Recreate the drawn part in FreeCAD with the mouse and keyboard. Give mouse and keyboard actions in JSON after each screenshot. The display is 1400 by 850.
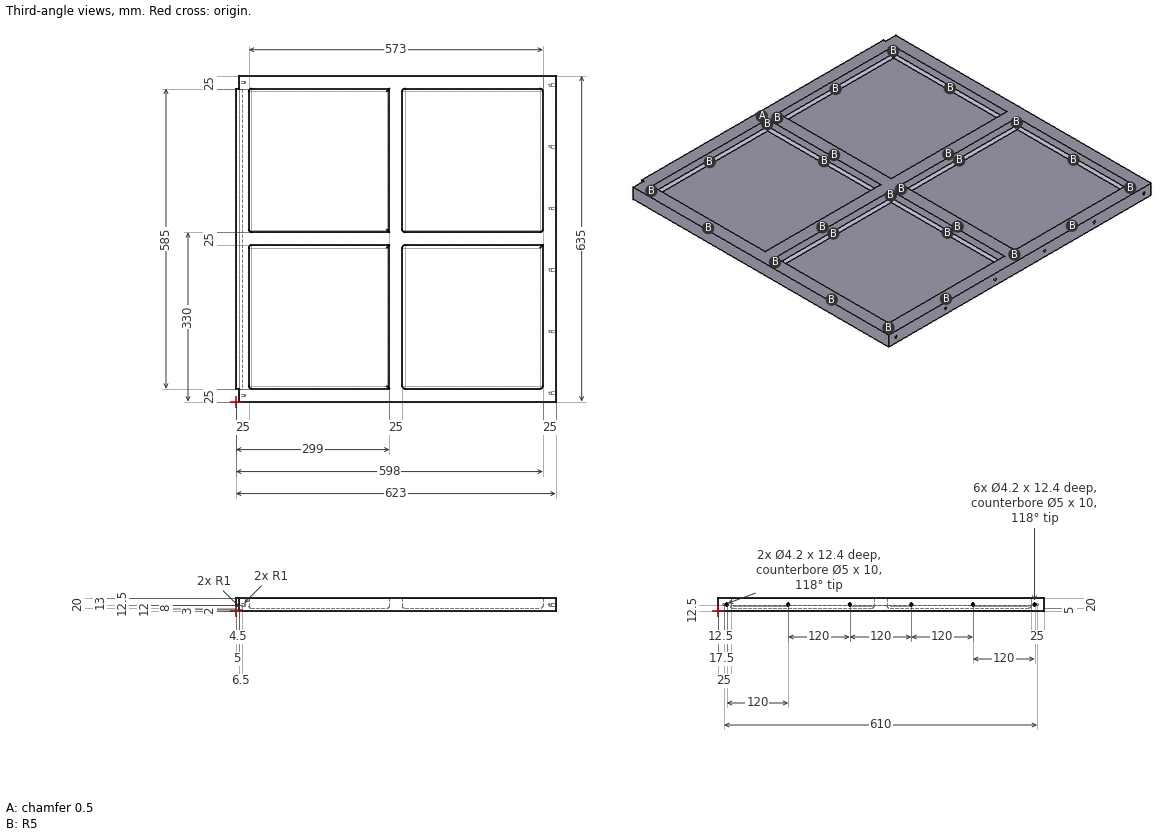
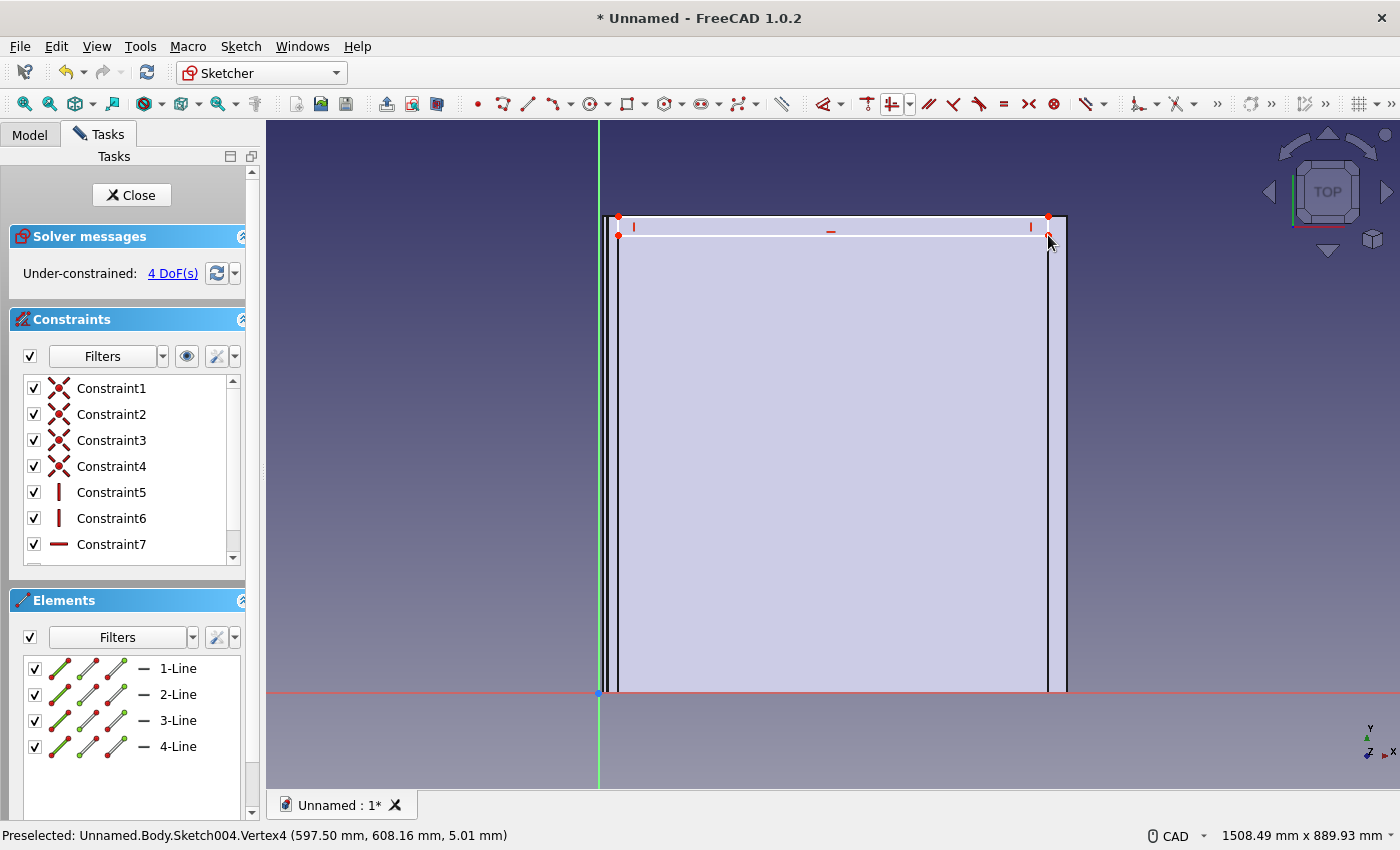
{"action": "left_click", "coordinate": [822, 104]}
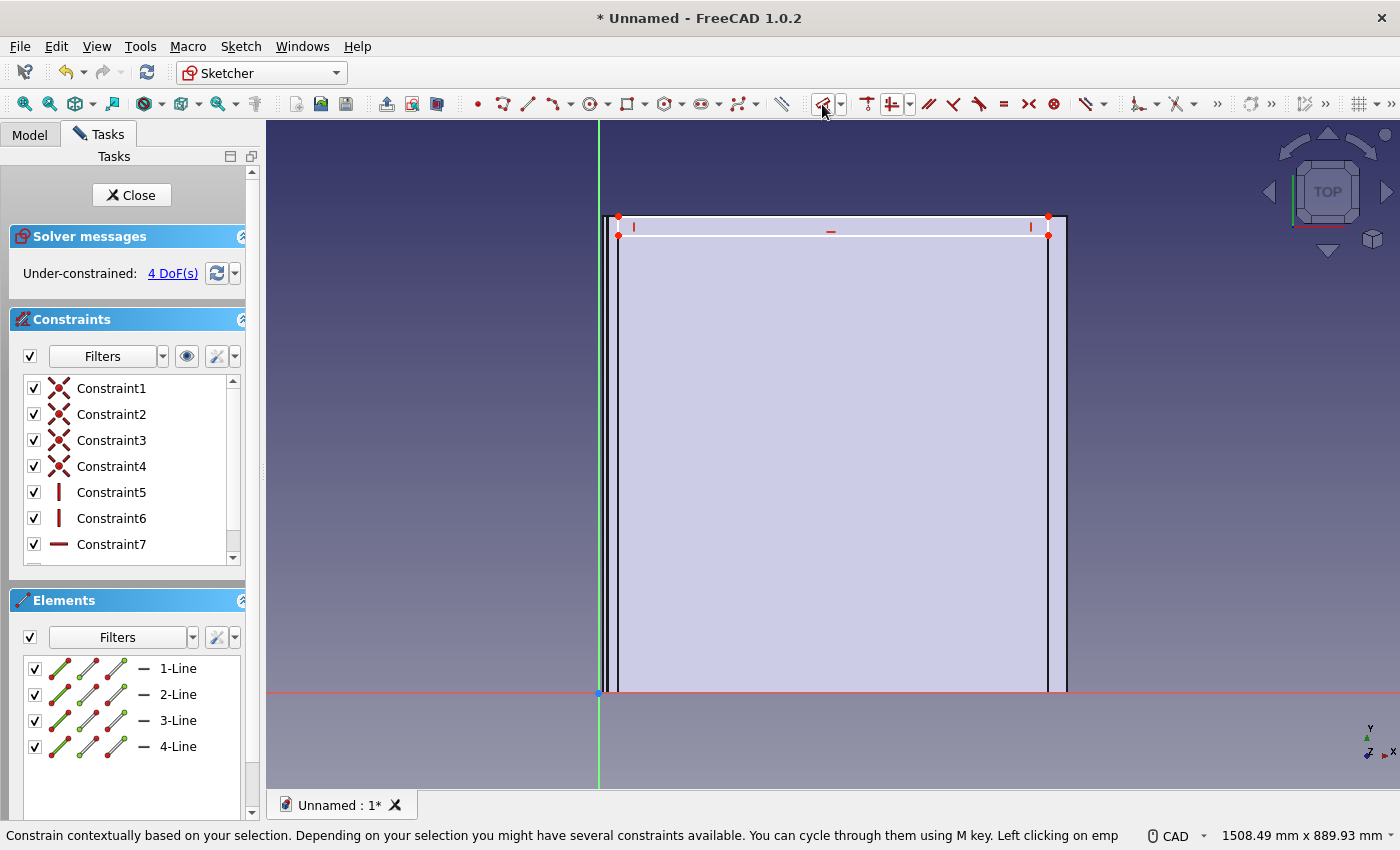
{"action": "scroll", "coordinate": [618, 227], "scroll_direction": "up", "scroll_amount": 4}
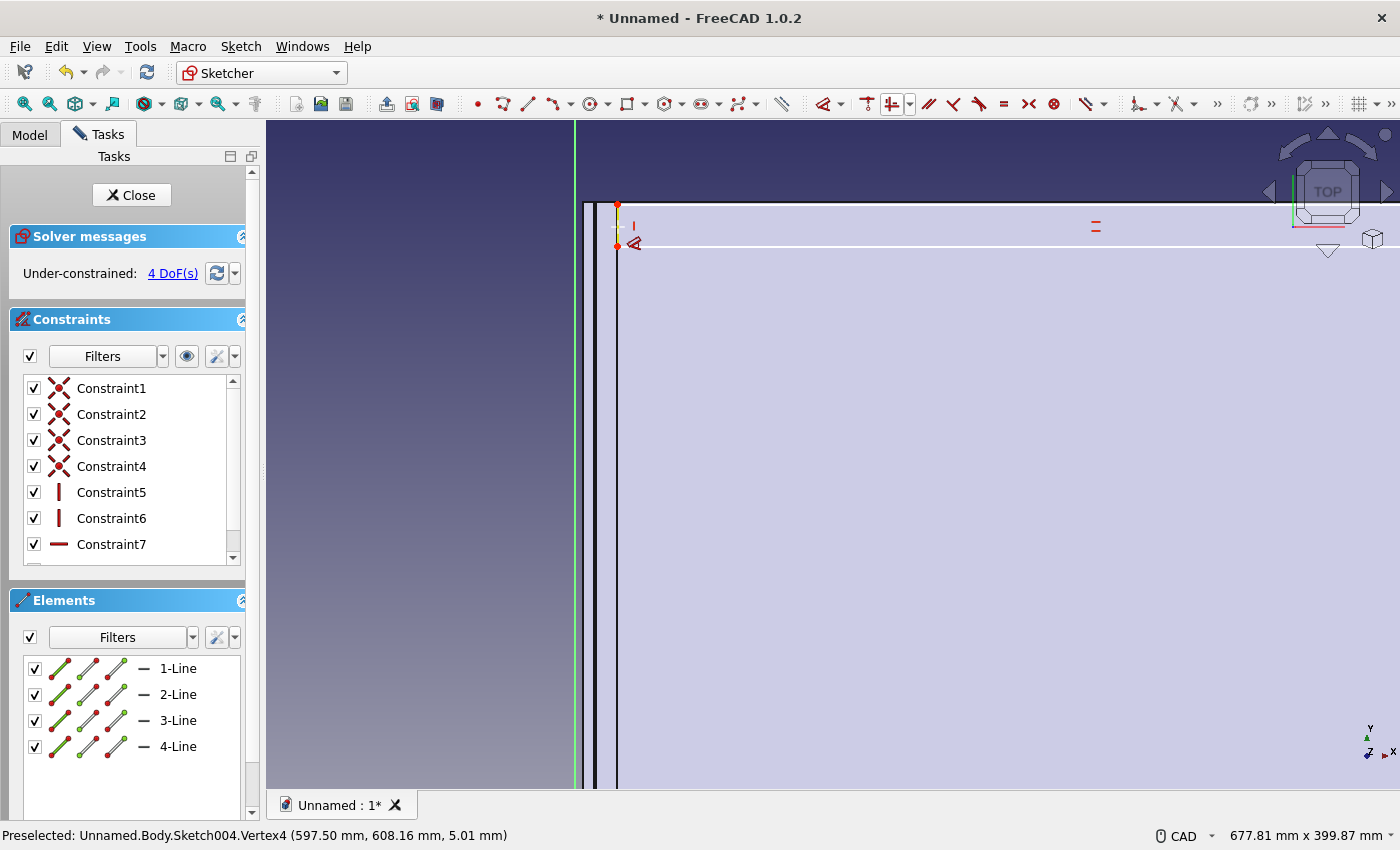
{"action": "left_click", "coordinate": [618, 226]}
{"action": "left_click", "coordinate": [652, 226]}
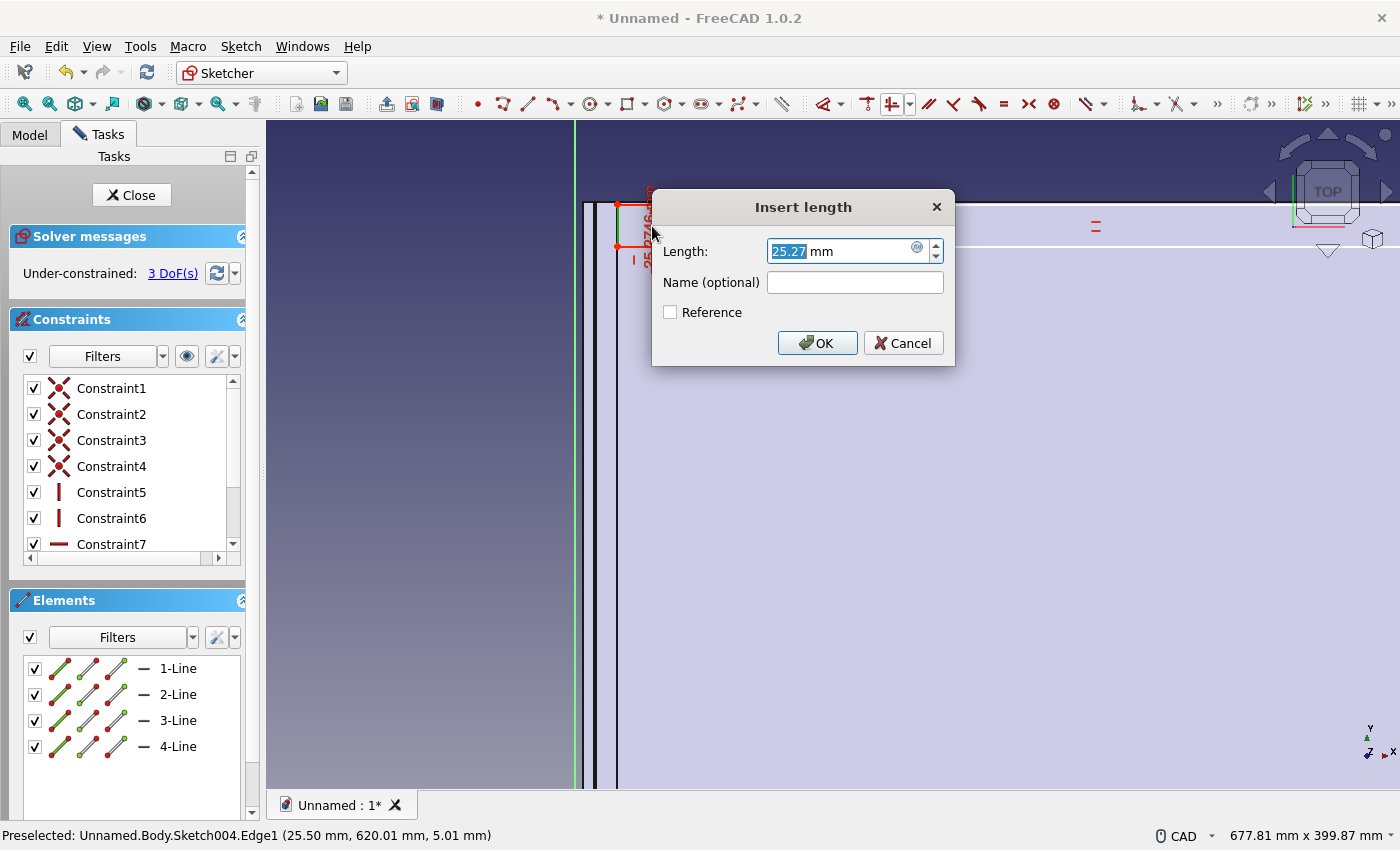
{"action": "type", "text": "25"}
{"action": "key", "text": "Return"}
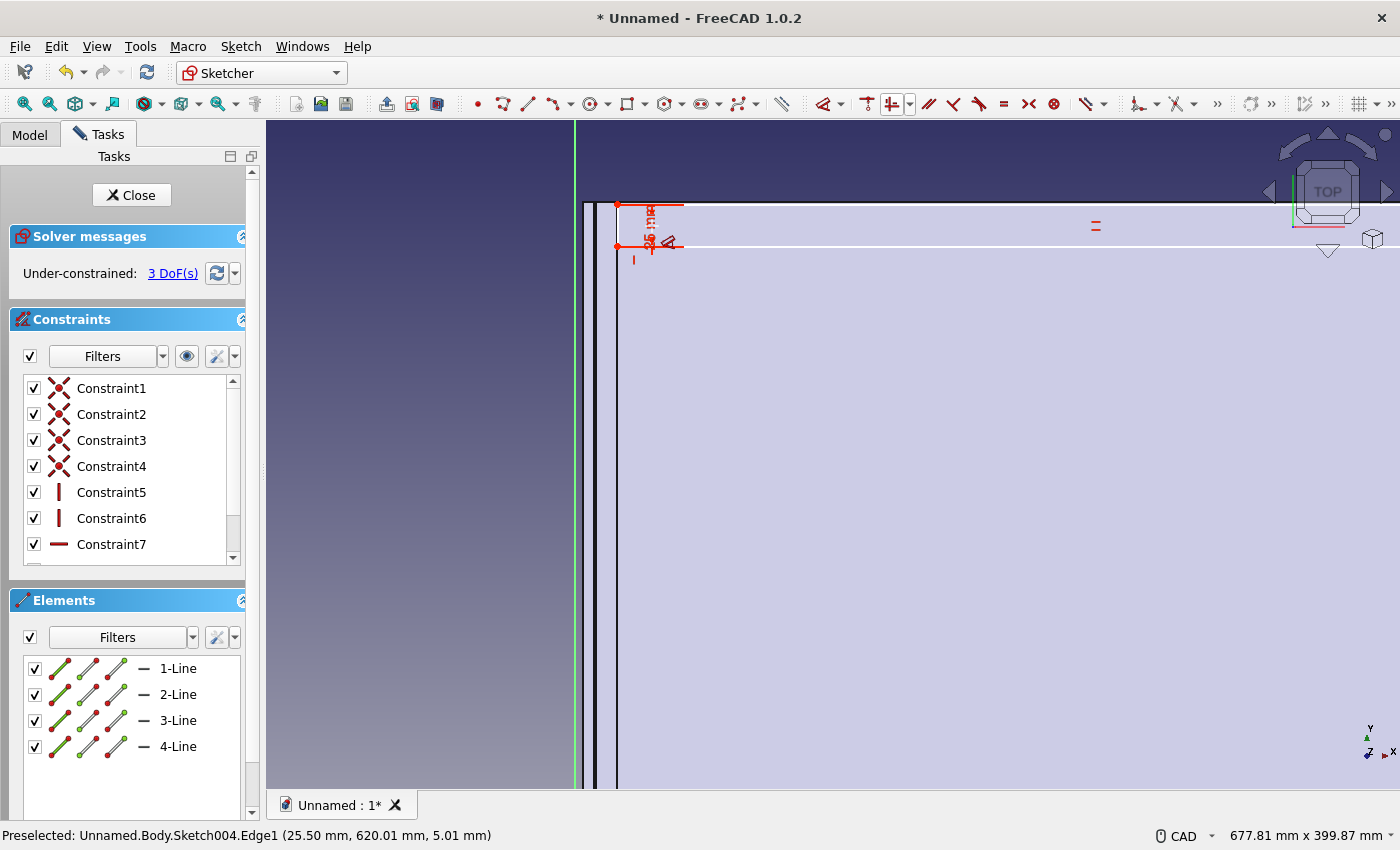
{"action": "left_click", "coordinate": [905, 247]}
{"action": "left_click", "coordinate": [926, 281]}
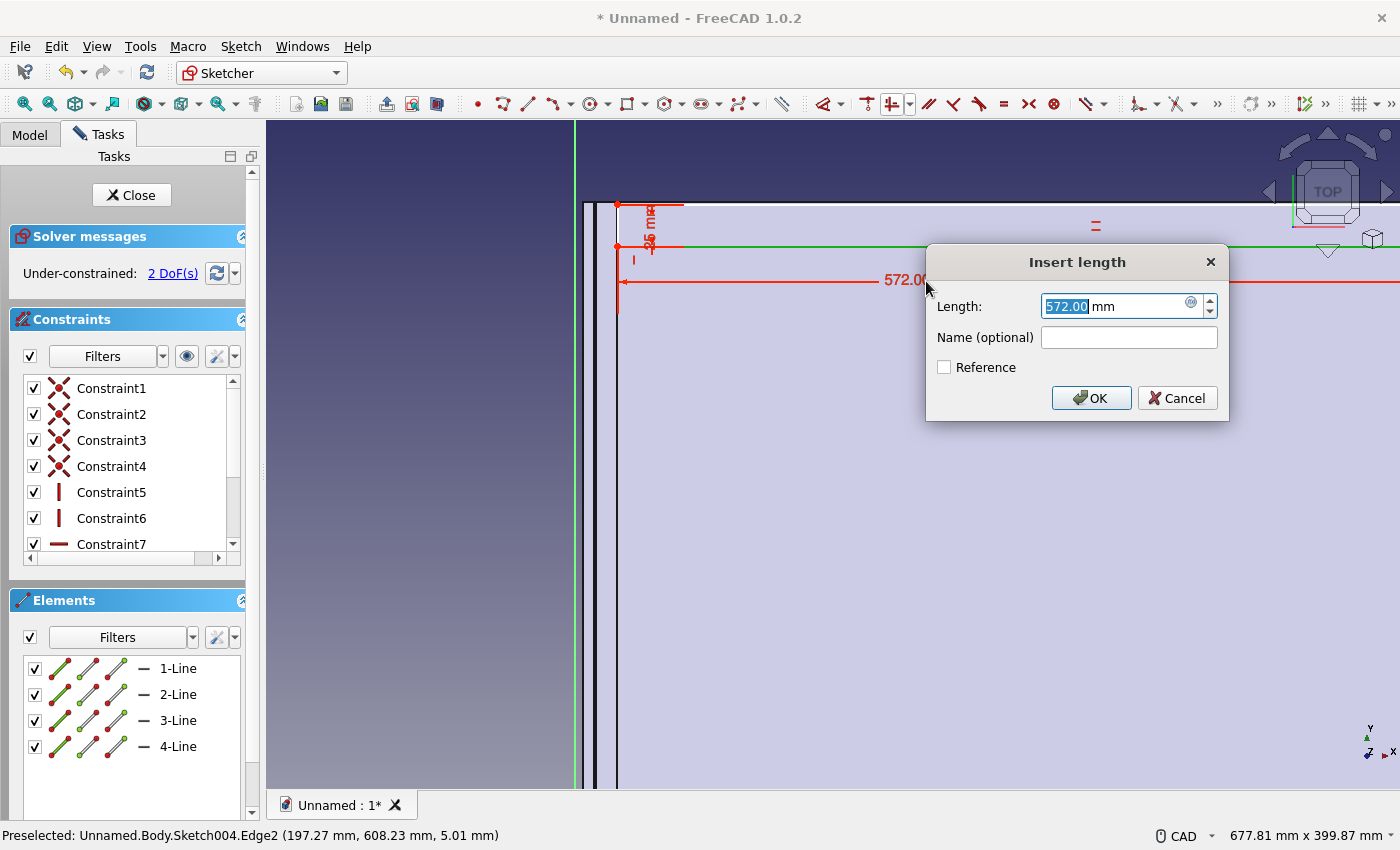
{"action": "type", "text": "573"}
{"action": "key", "text": "Return"}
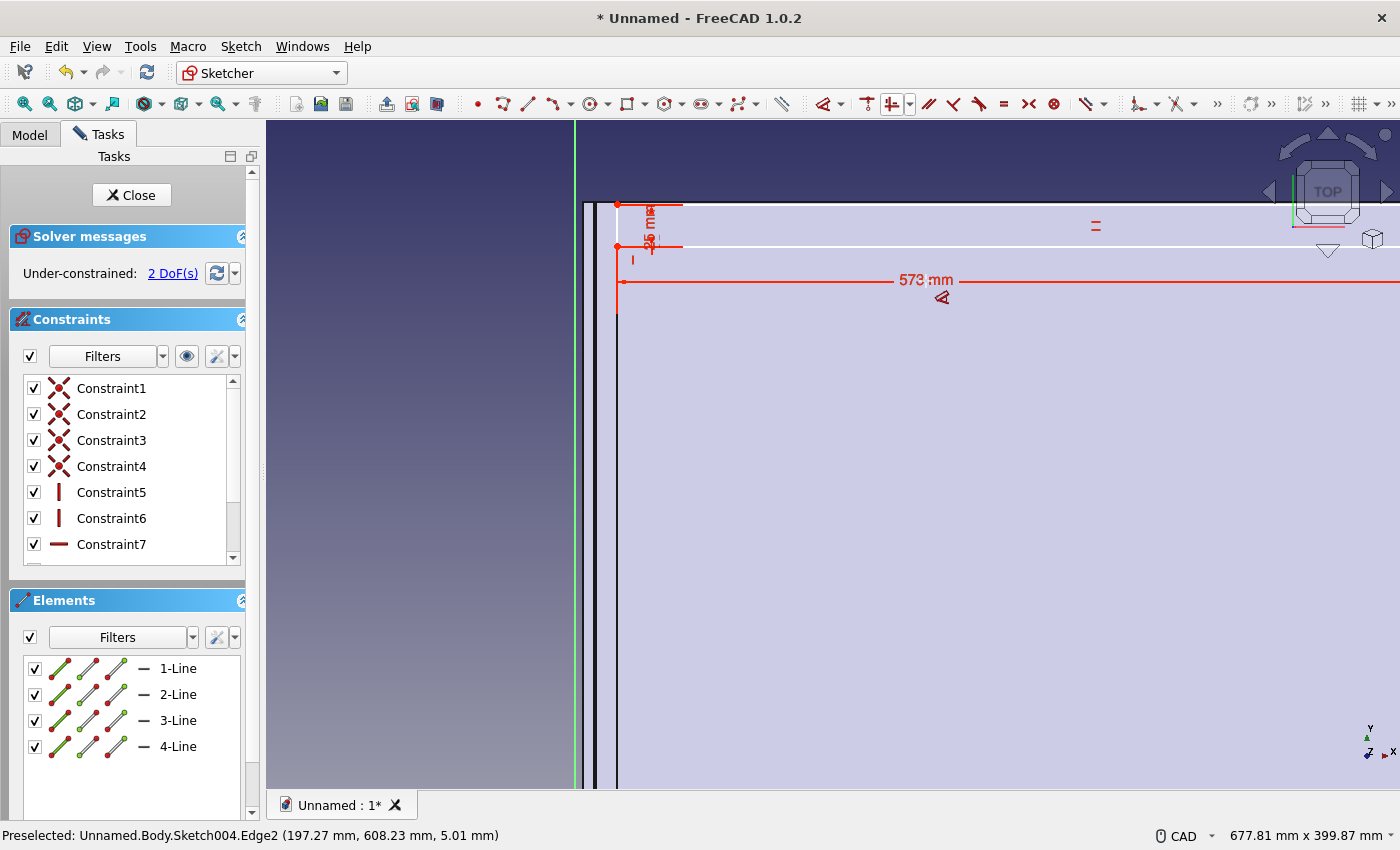
{"action": "left_click", "coordinate": [617, 205]}
{"action": "left_click", "coordinate": [596, 171]}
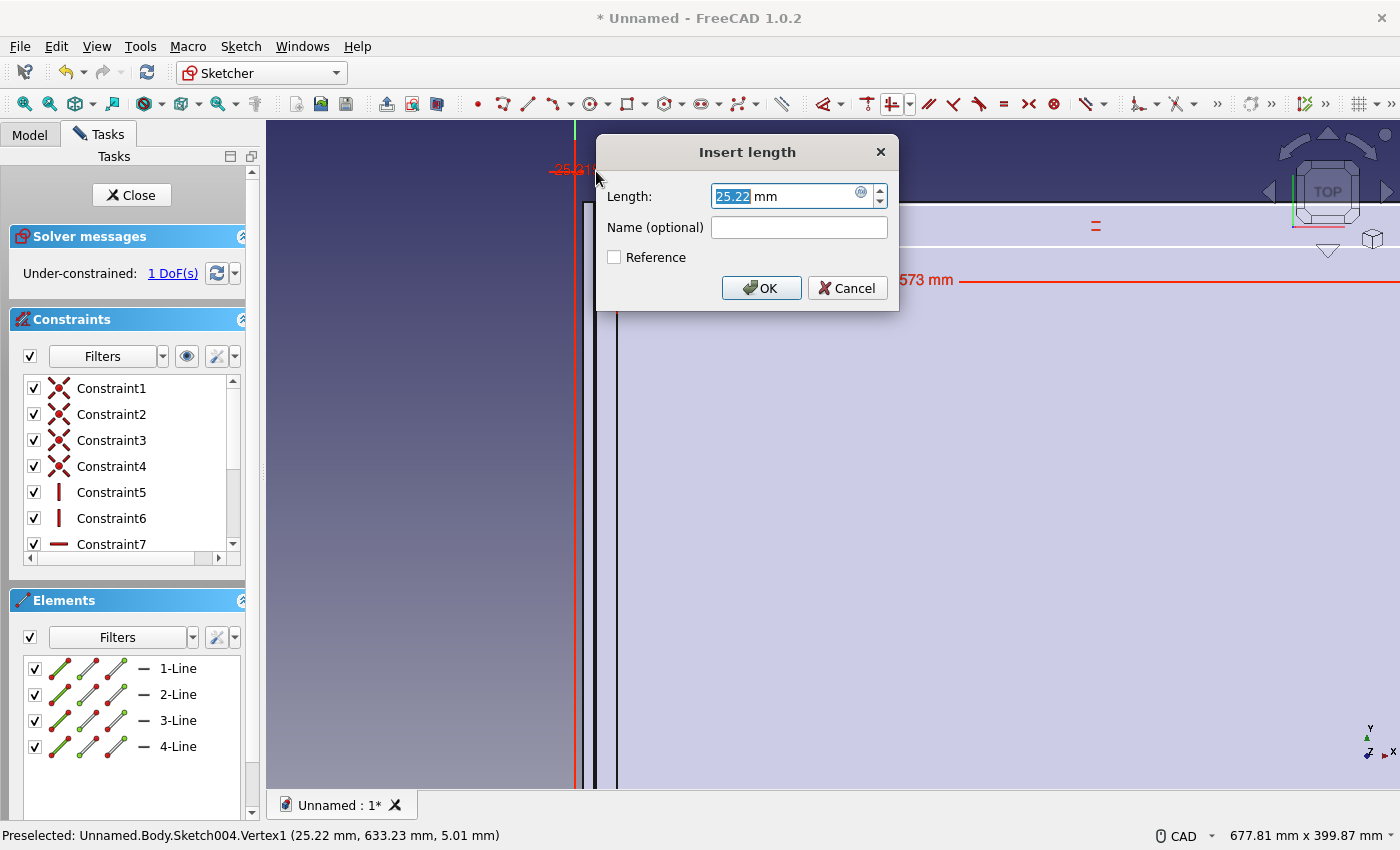
{"action": "type", "text": "25"}
{"action": "key", "text": "Return"}